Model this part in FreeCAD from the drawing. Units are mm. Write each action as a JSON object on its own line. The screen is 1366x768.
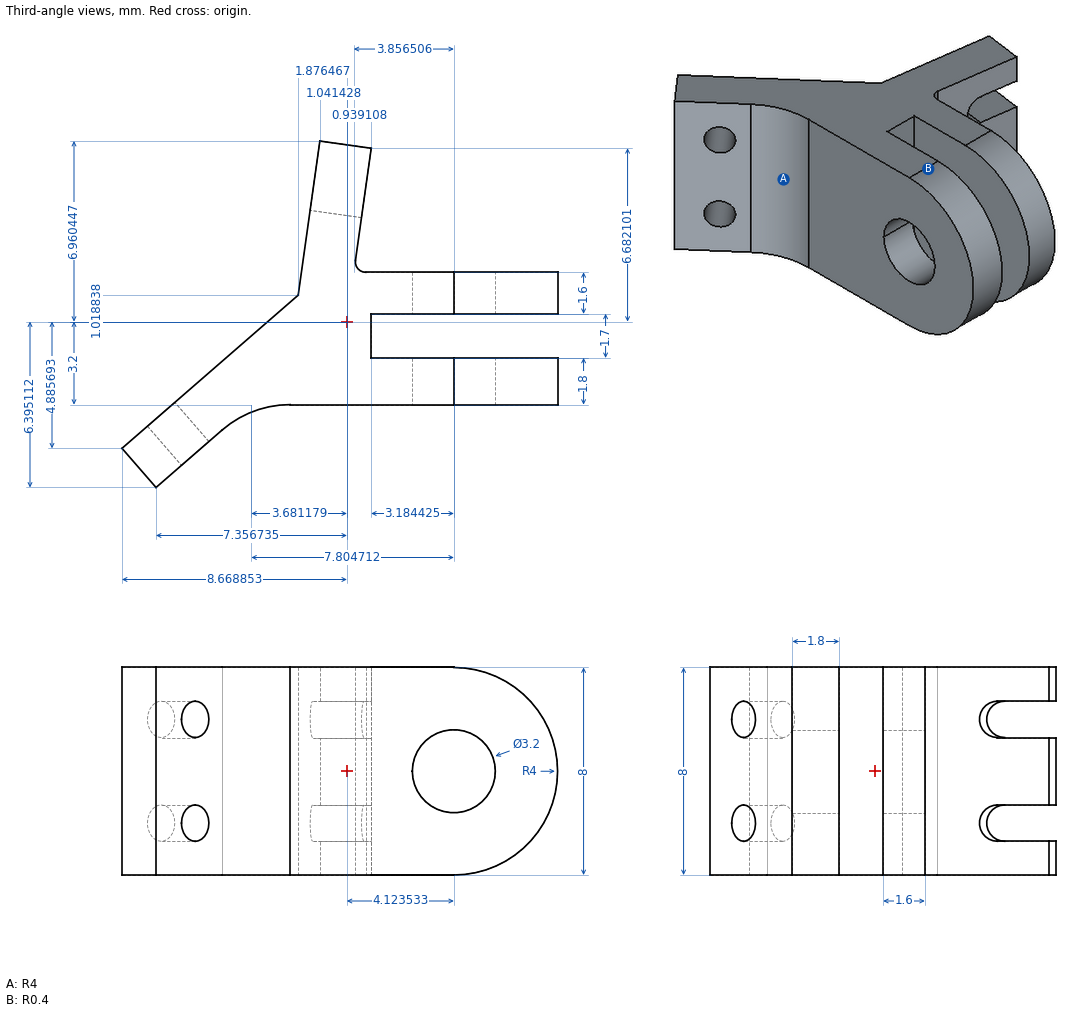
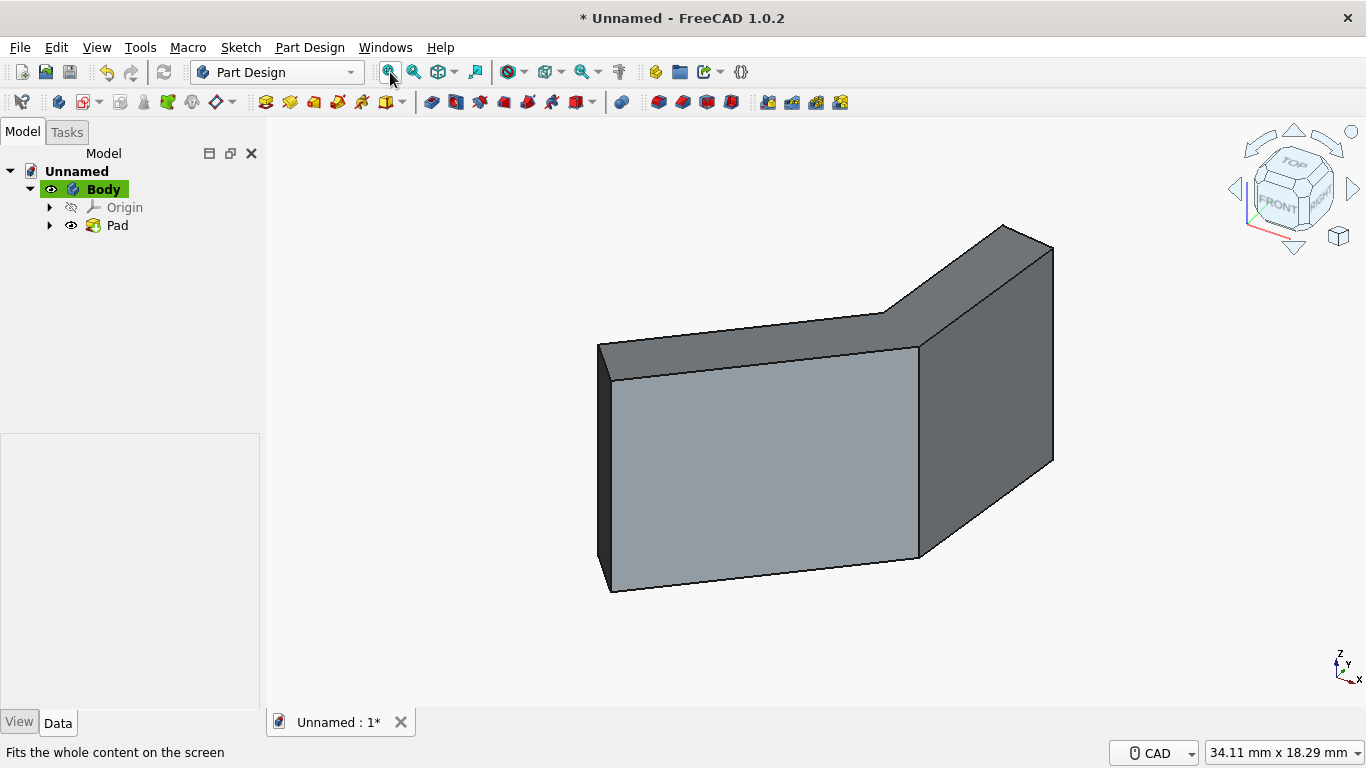
{"action": "key", "text": "6"}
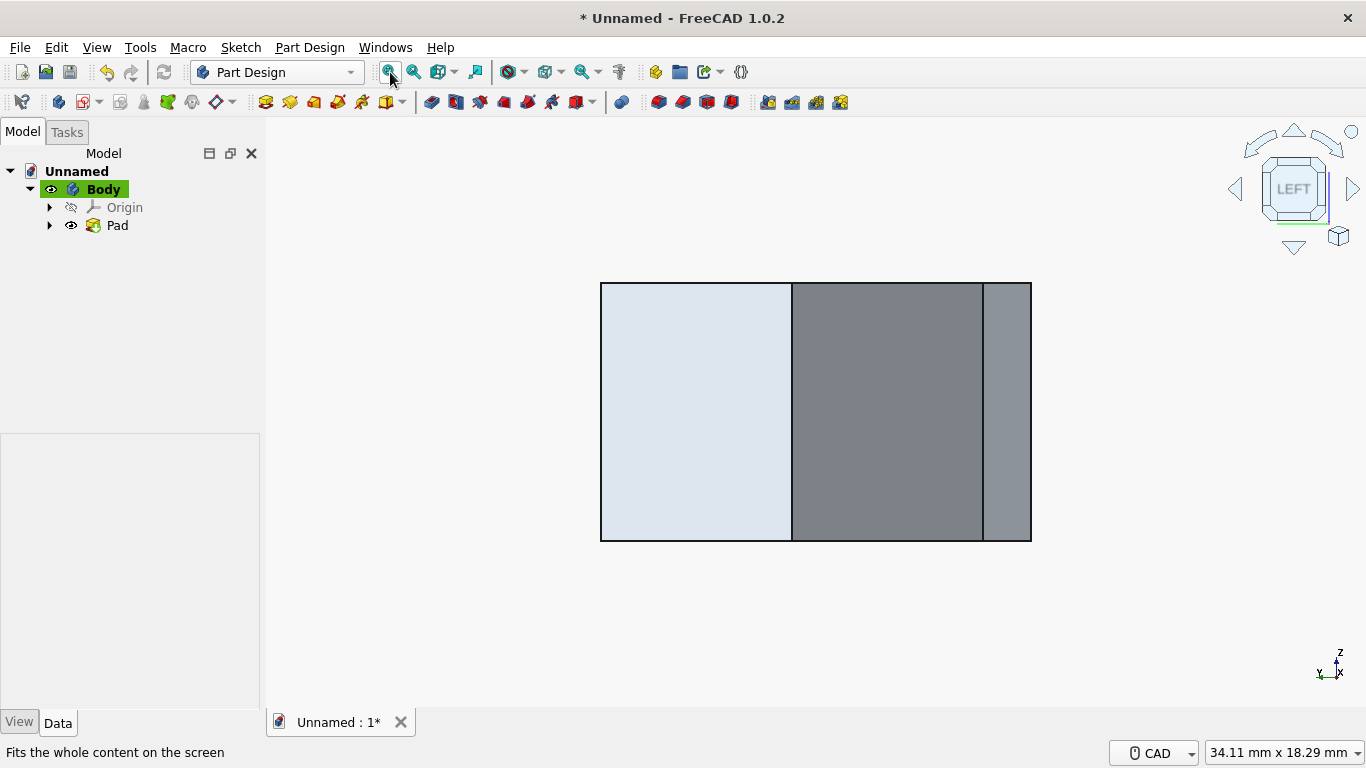
{"action": "left_click", "coordinate": [390, 72]}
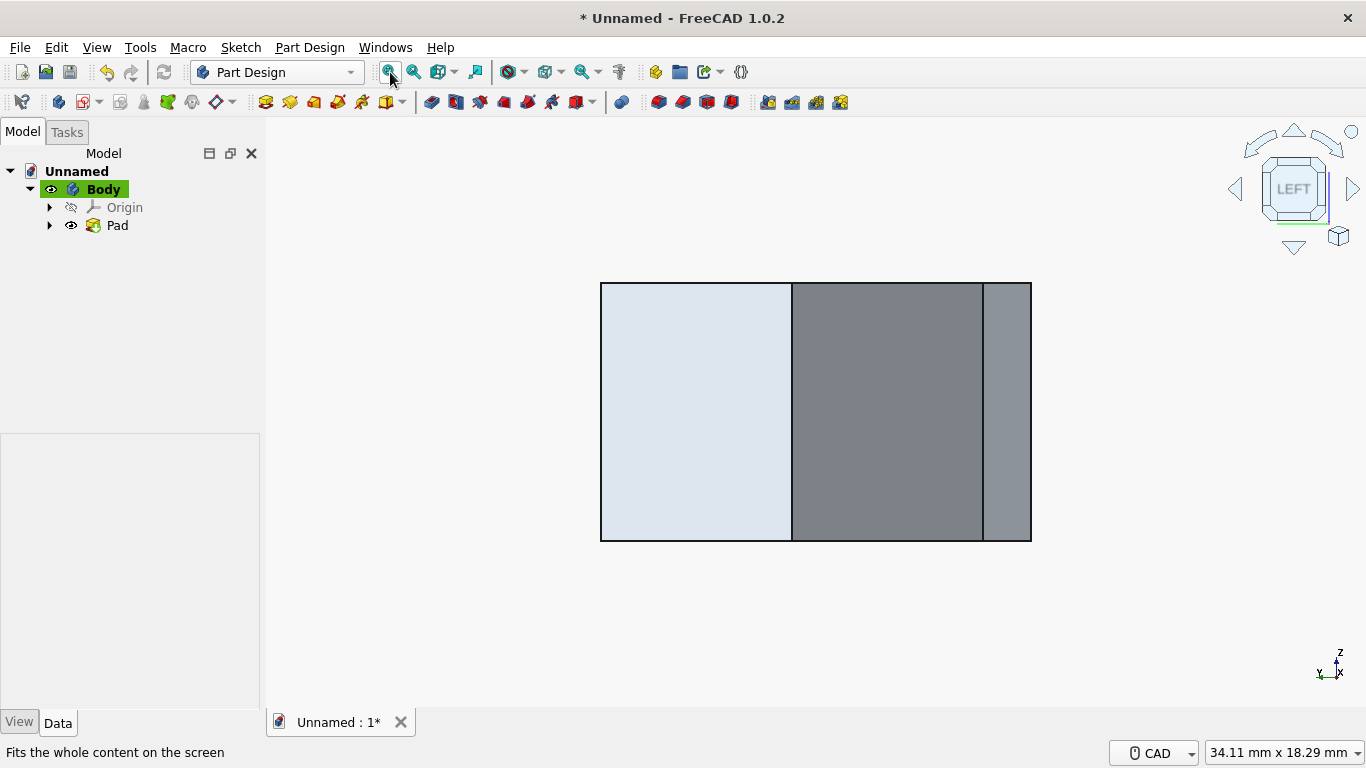
{"action": "left_click", "coordinate": [696, 411]}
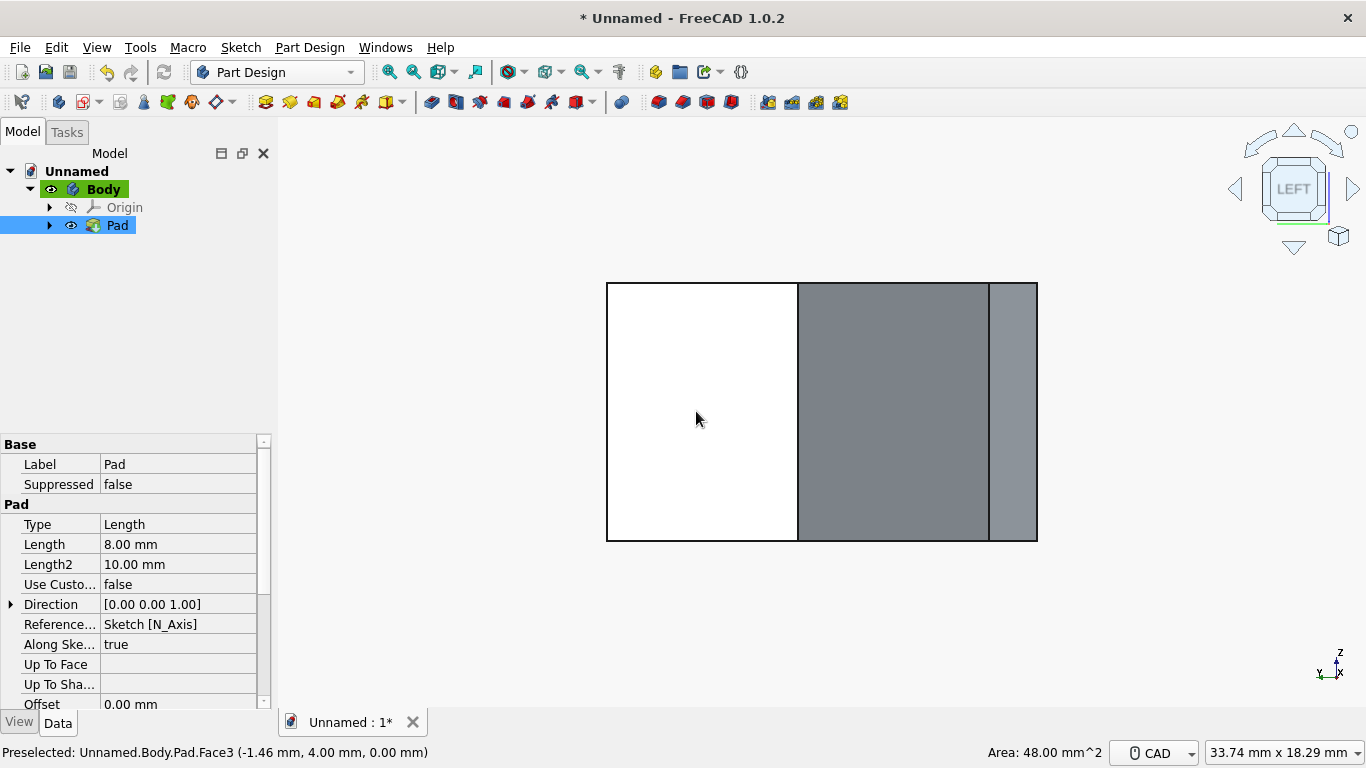
{"action": "left_click", "coordinate": [84, 102]}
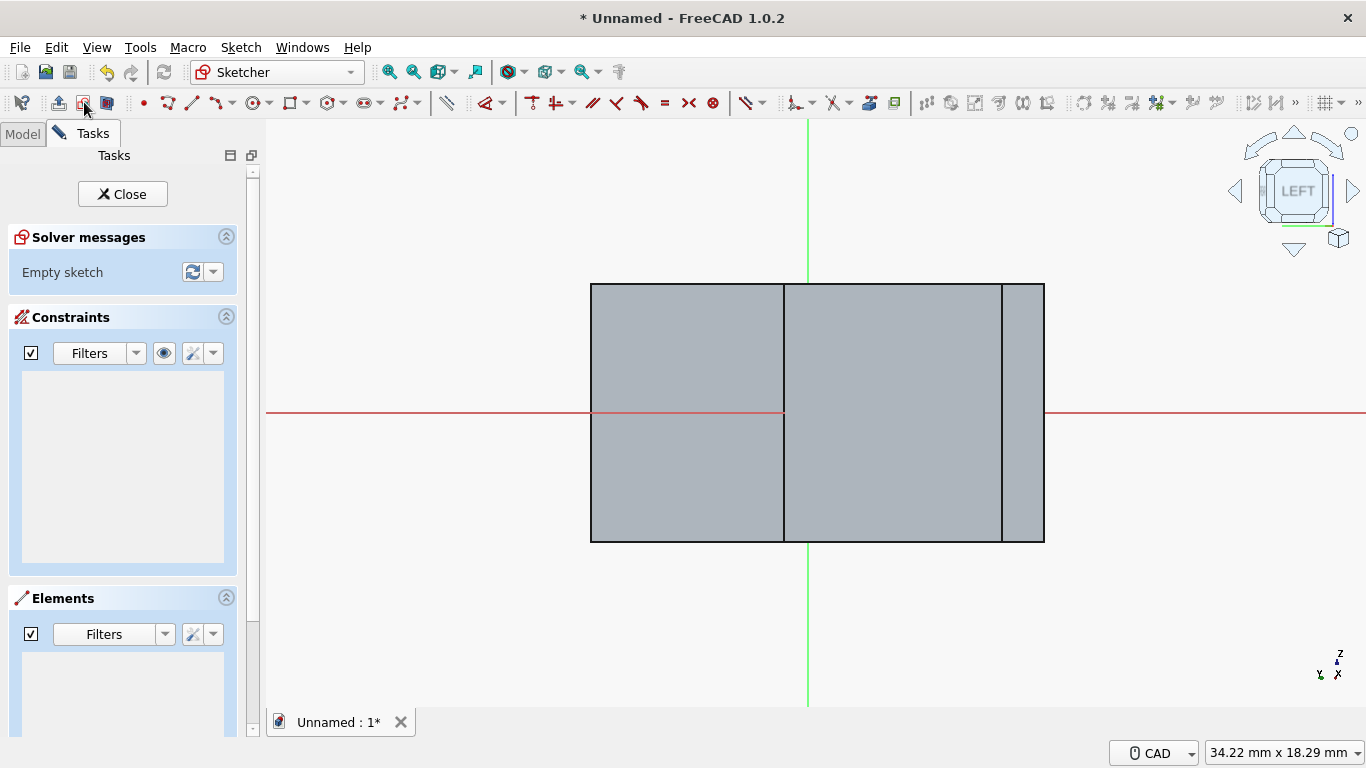
{"action": "scroll", "coordinate": [660, 413], "scroll_direction": "up", "scroll_amount": 4}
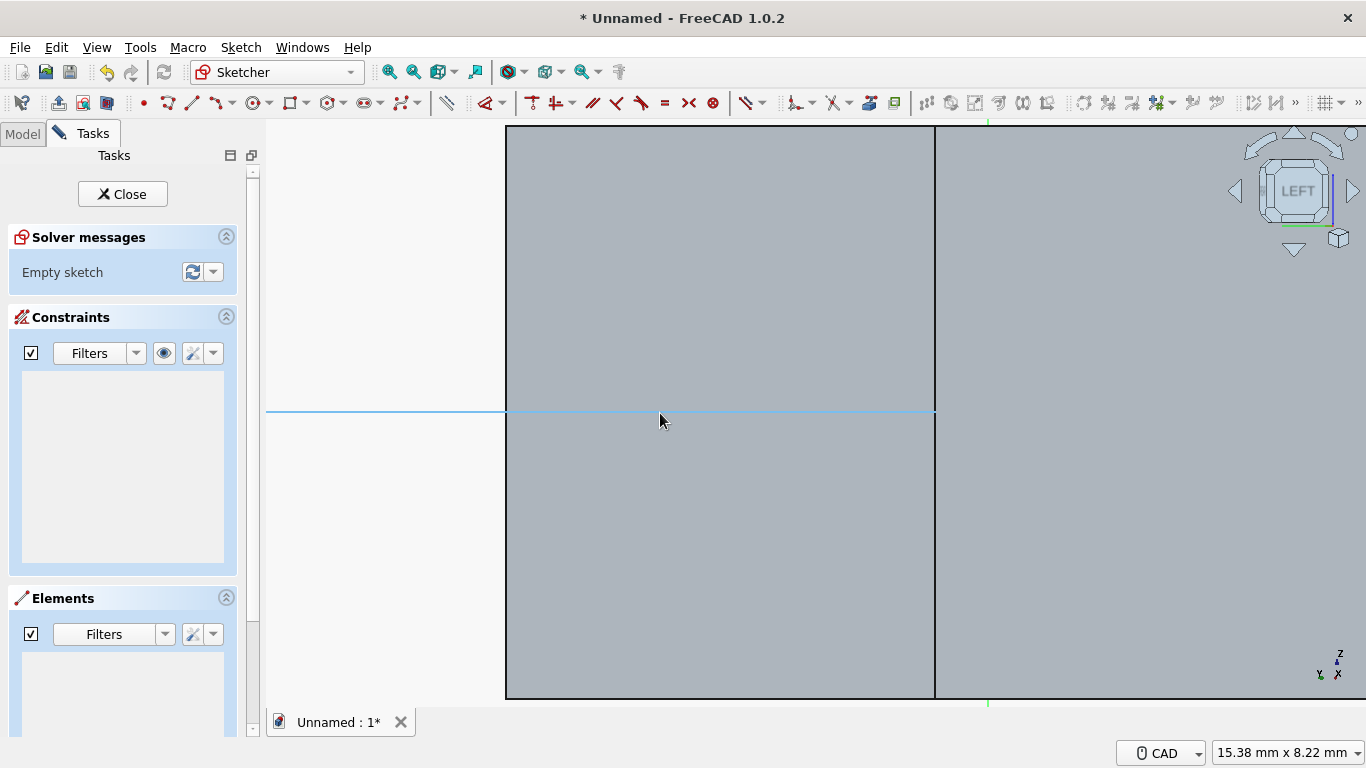
{"action": "left_click", "coordinate": [168, 104]}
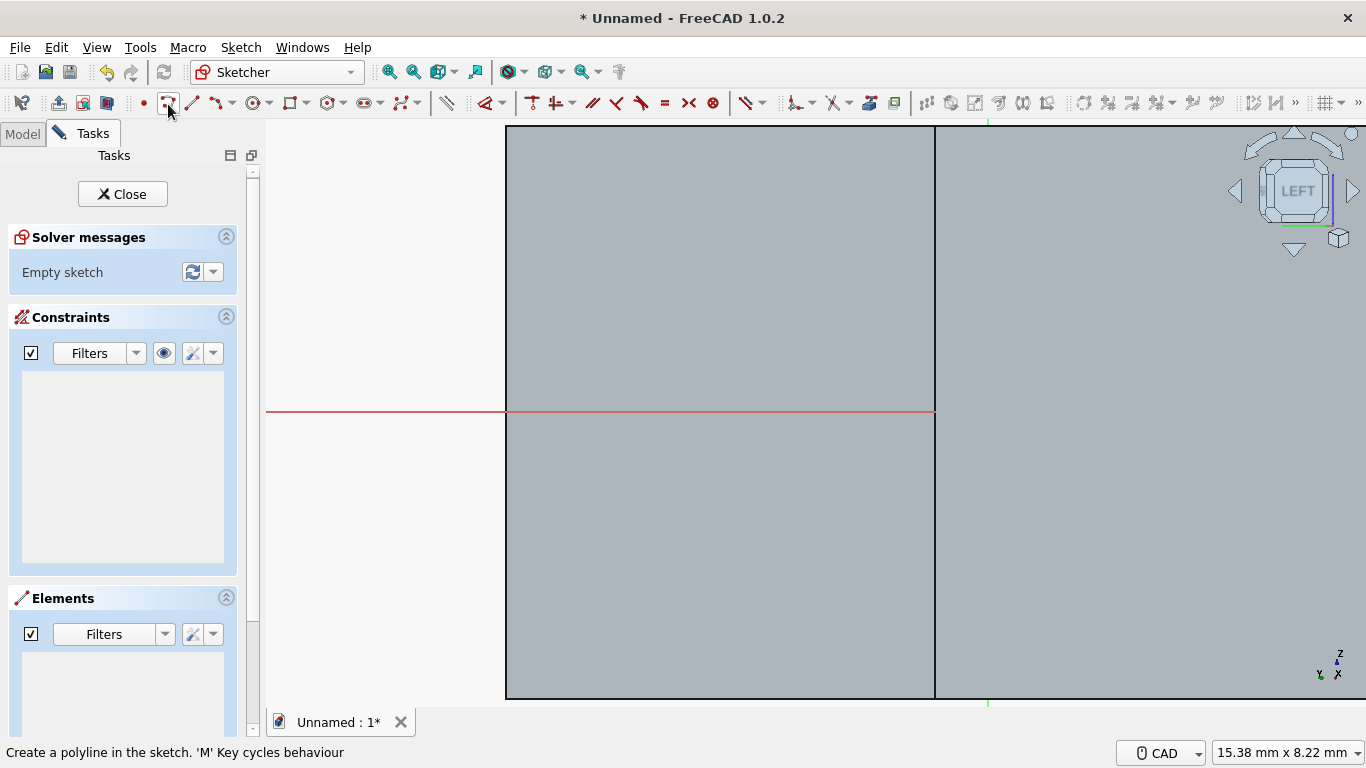
{"action": "left_click", "coordinate": [649, 505]}
{"action": "left_click", "coordinate": [506, 505]}
{"action": "left_click", "coordinate": [506, 606]}
{"action": "left_click", "coordinate": [649, 606]}
{"action": "right_click", "coordinate": [649, 606]}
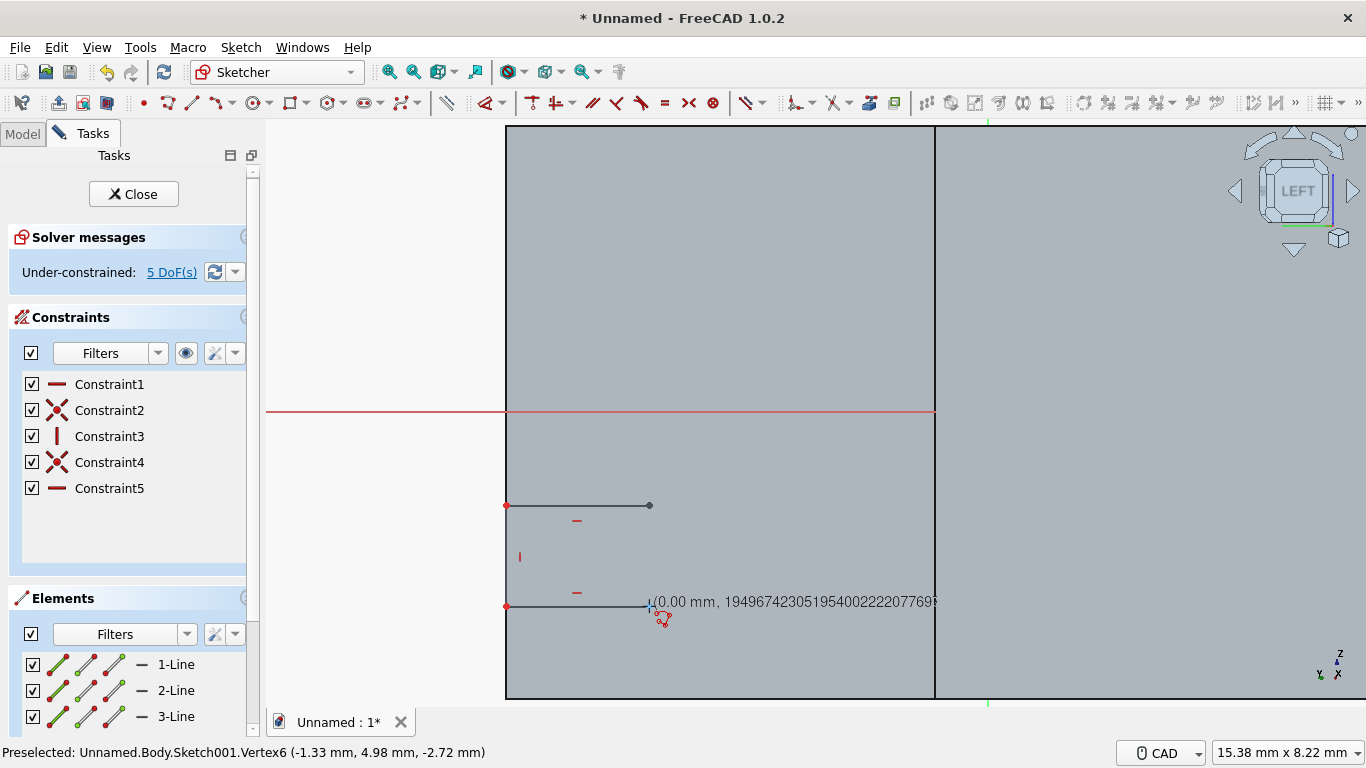
{"action": "left_click", "coordinate": [216, 104]}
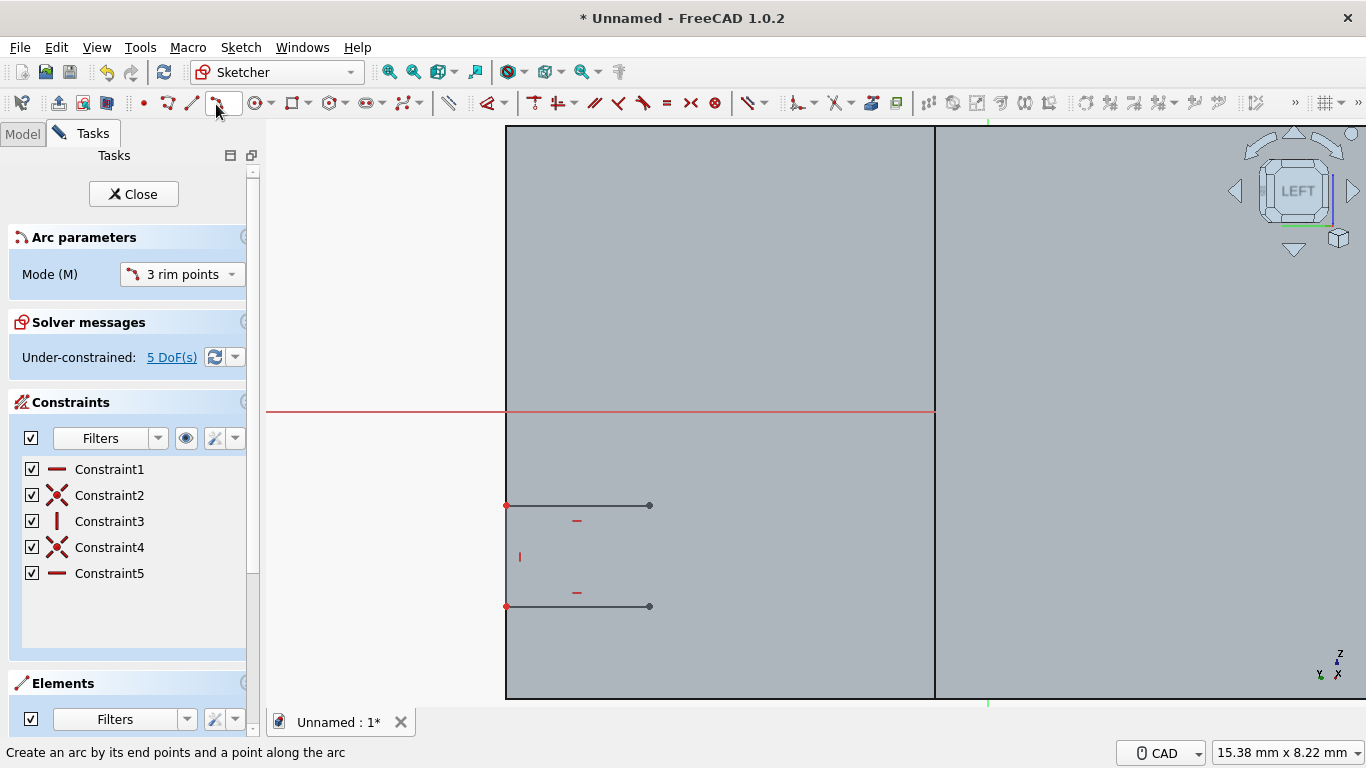
{"action": "left_click", "coordinate": [649, 607]}
{"action": "left_click", "coordinate": [649, 506]}
{"action": "left_click", "coordinate": [699, 555]}